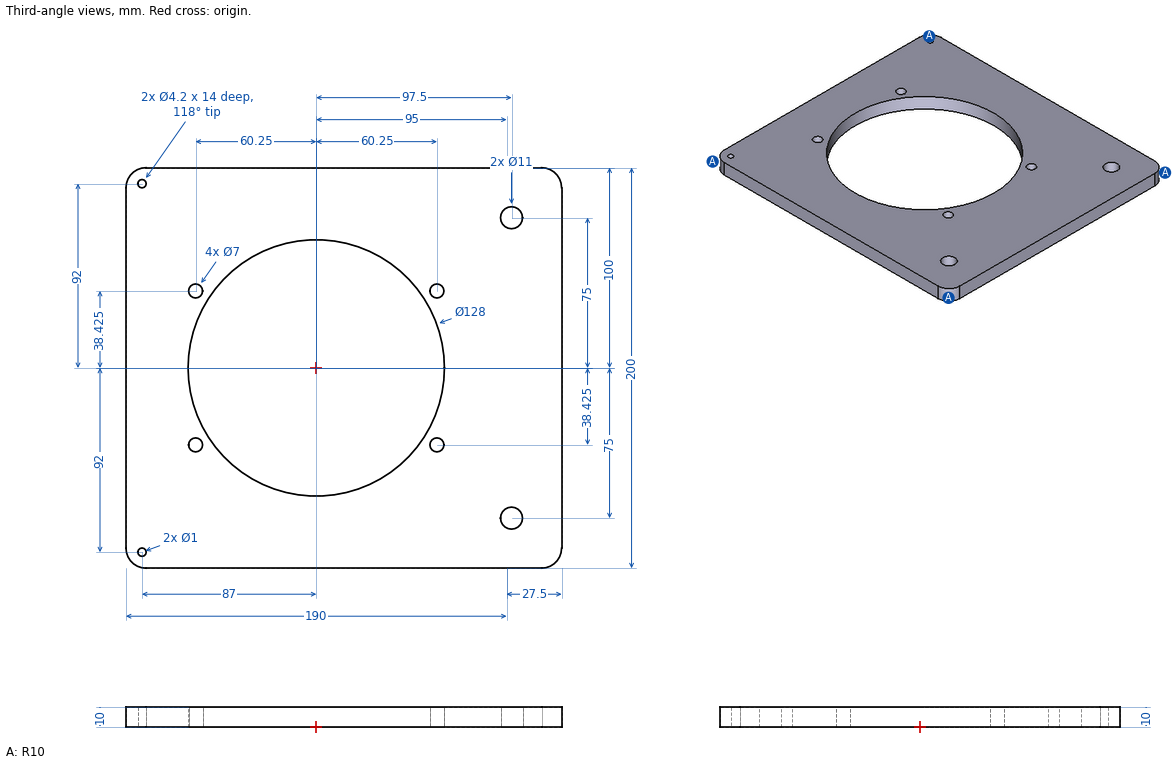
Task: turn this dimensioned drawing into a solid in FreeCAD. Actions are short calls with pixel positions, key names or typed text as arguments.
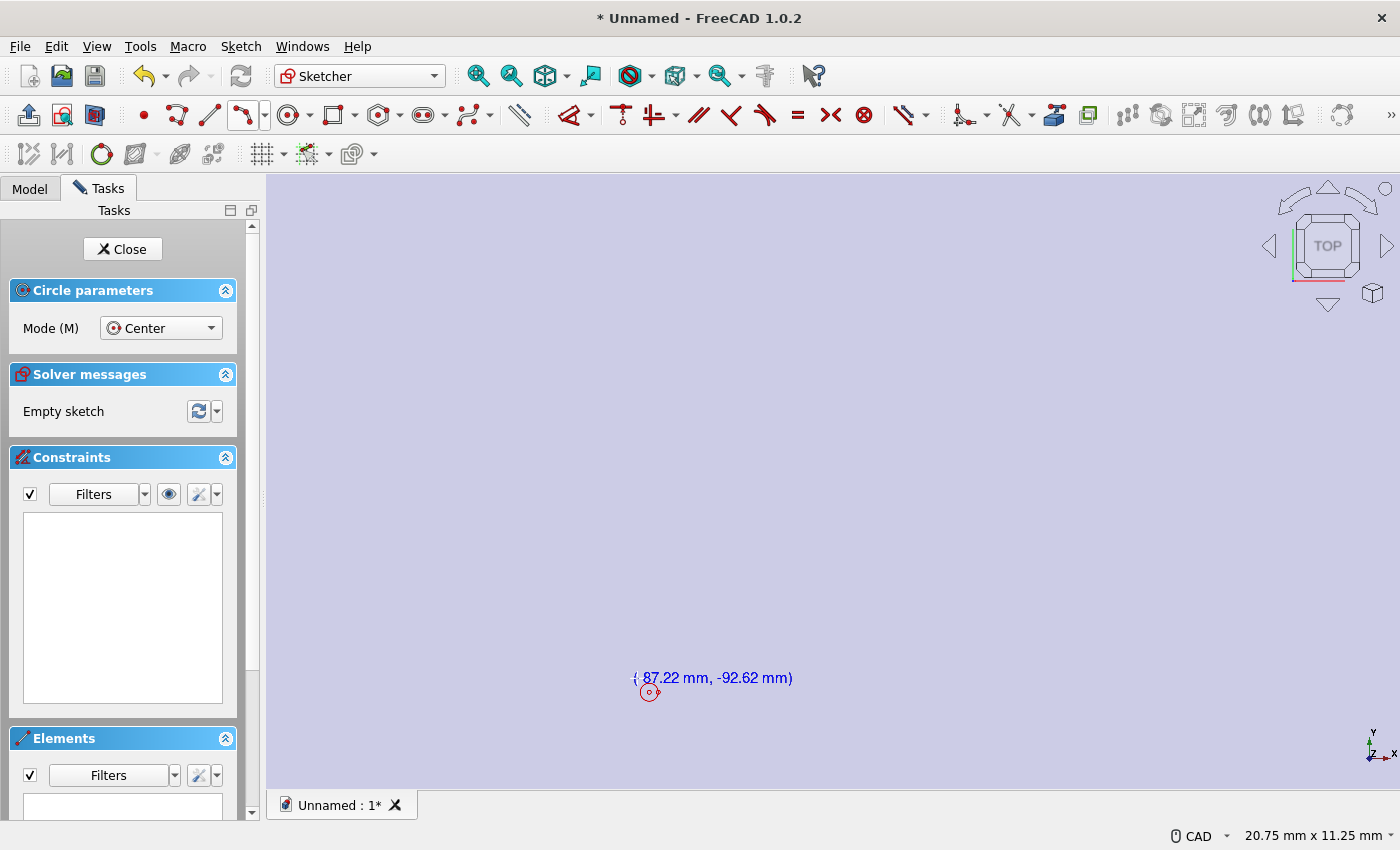
scroll(647, 736, down, 15)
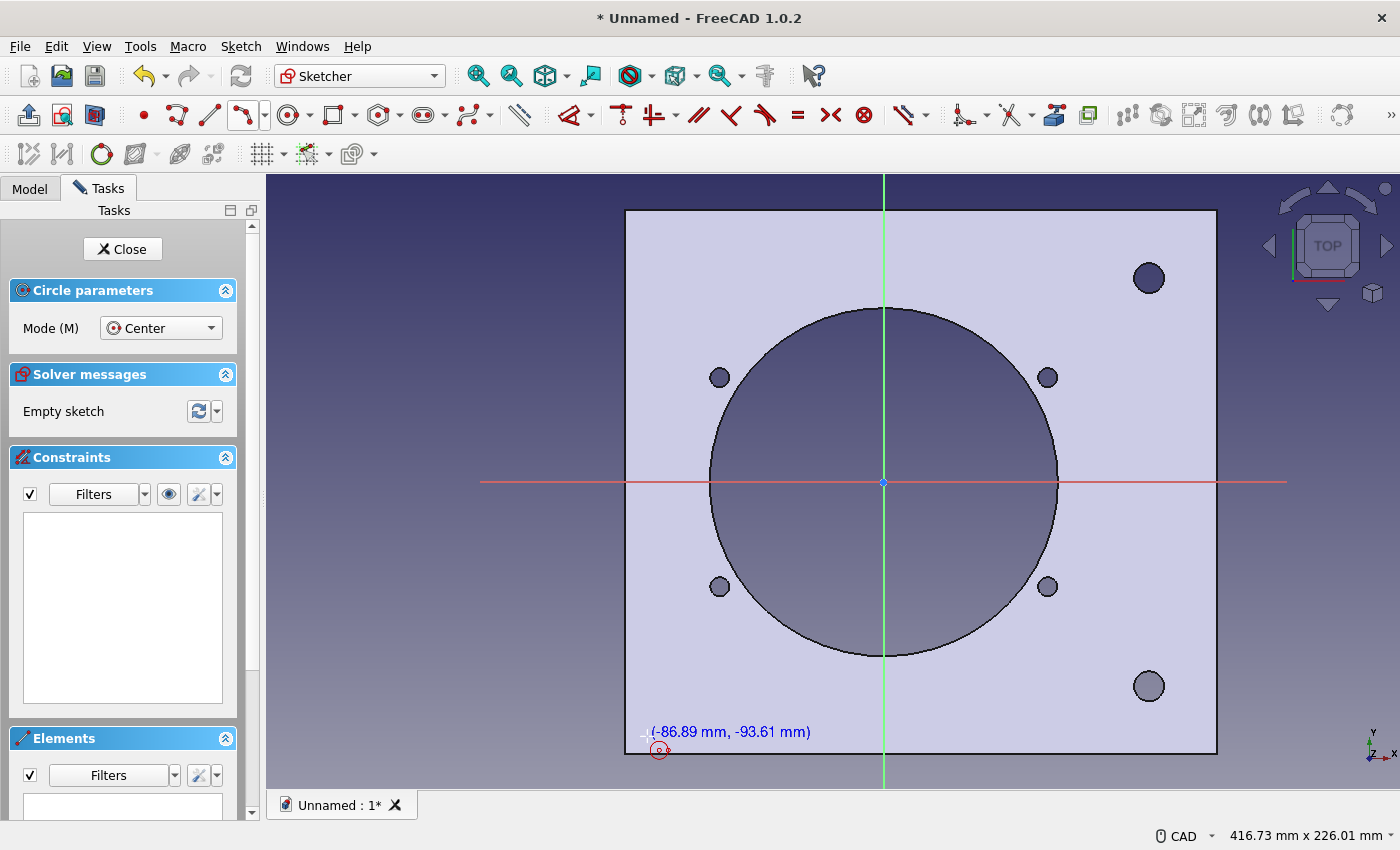
click(647, 733)
move(648, 732)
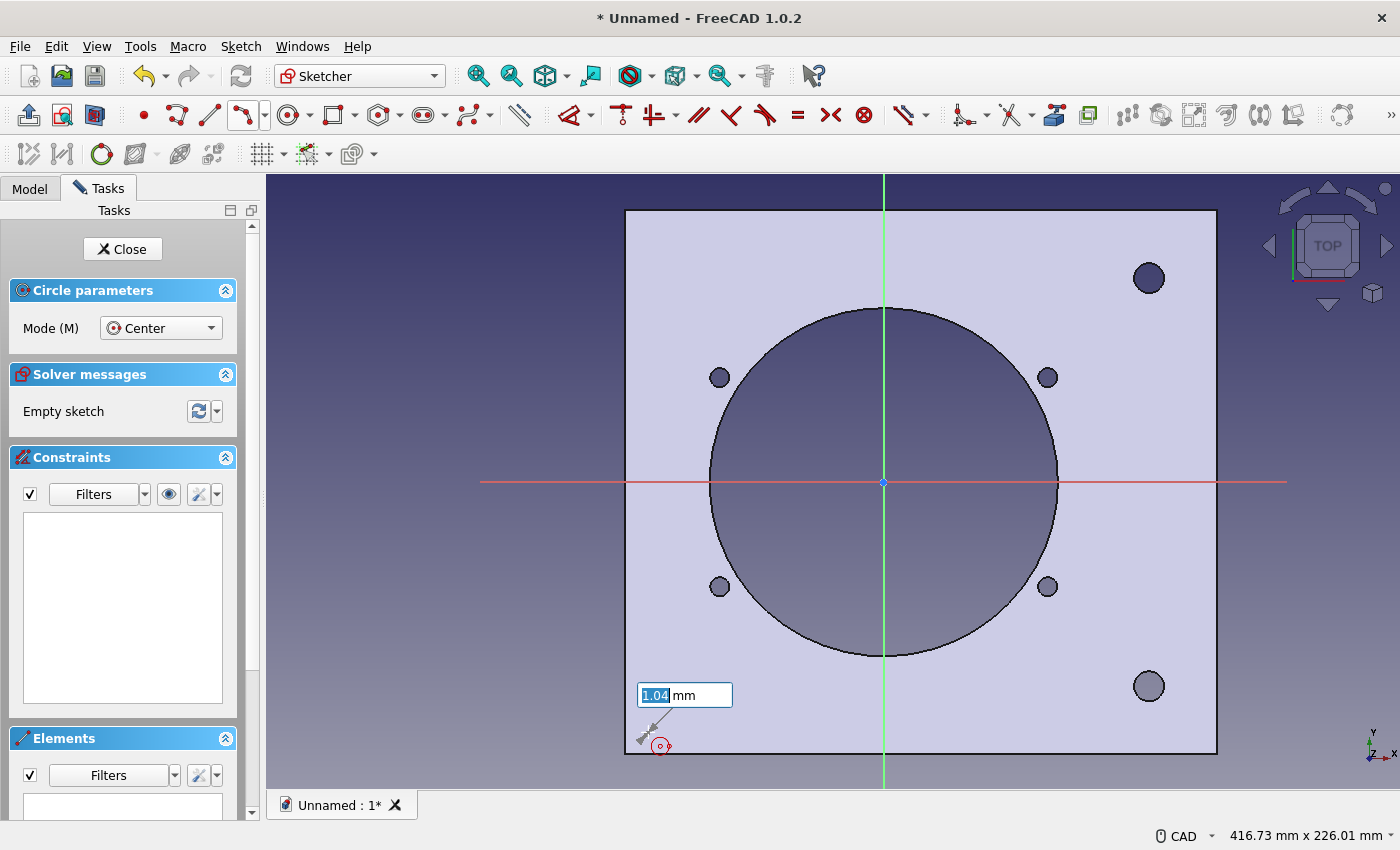
text(1)
key(Return)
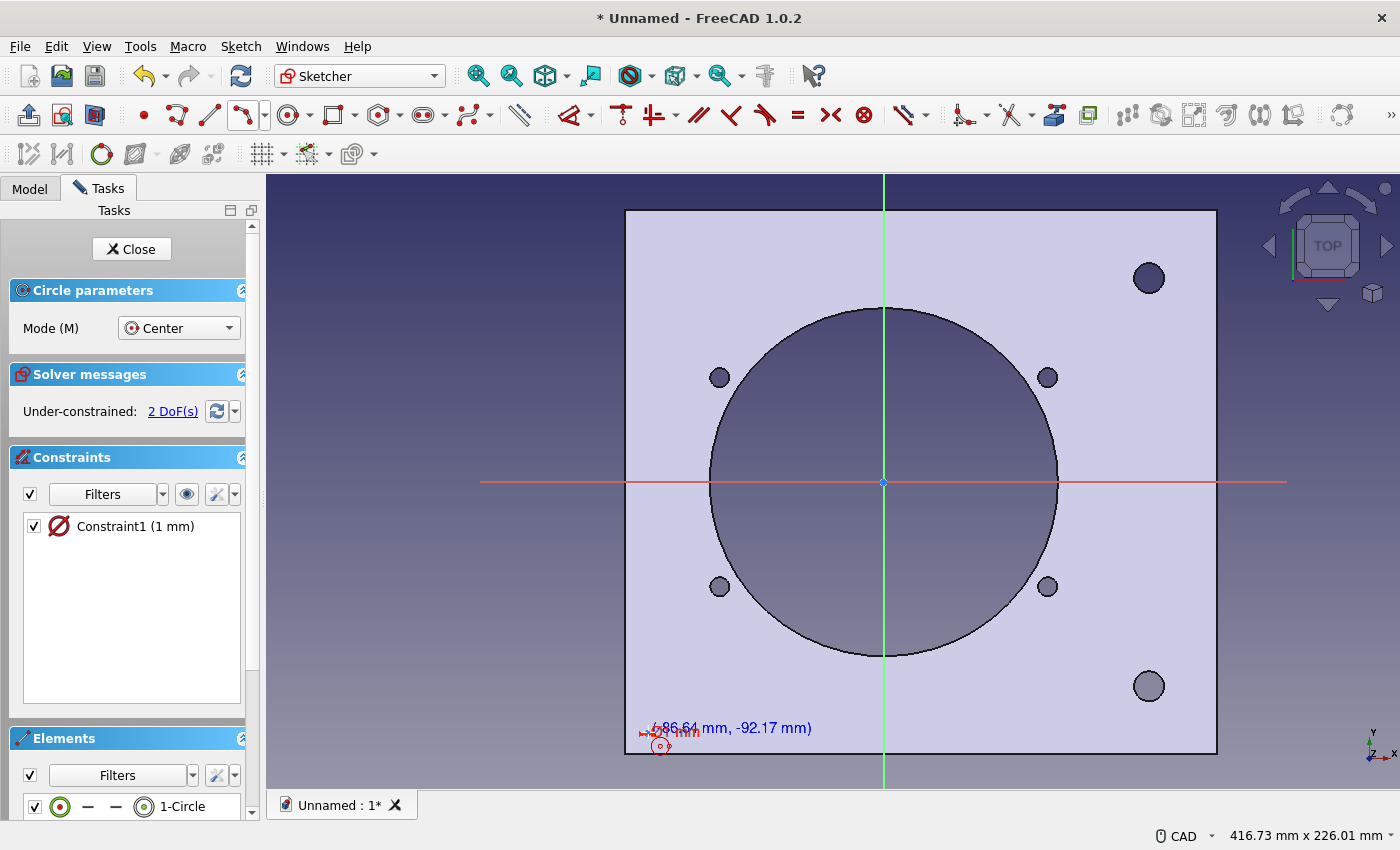
scroll(647, 232, up, 15)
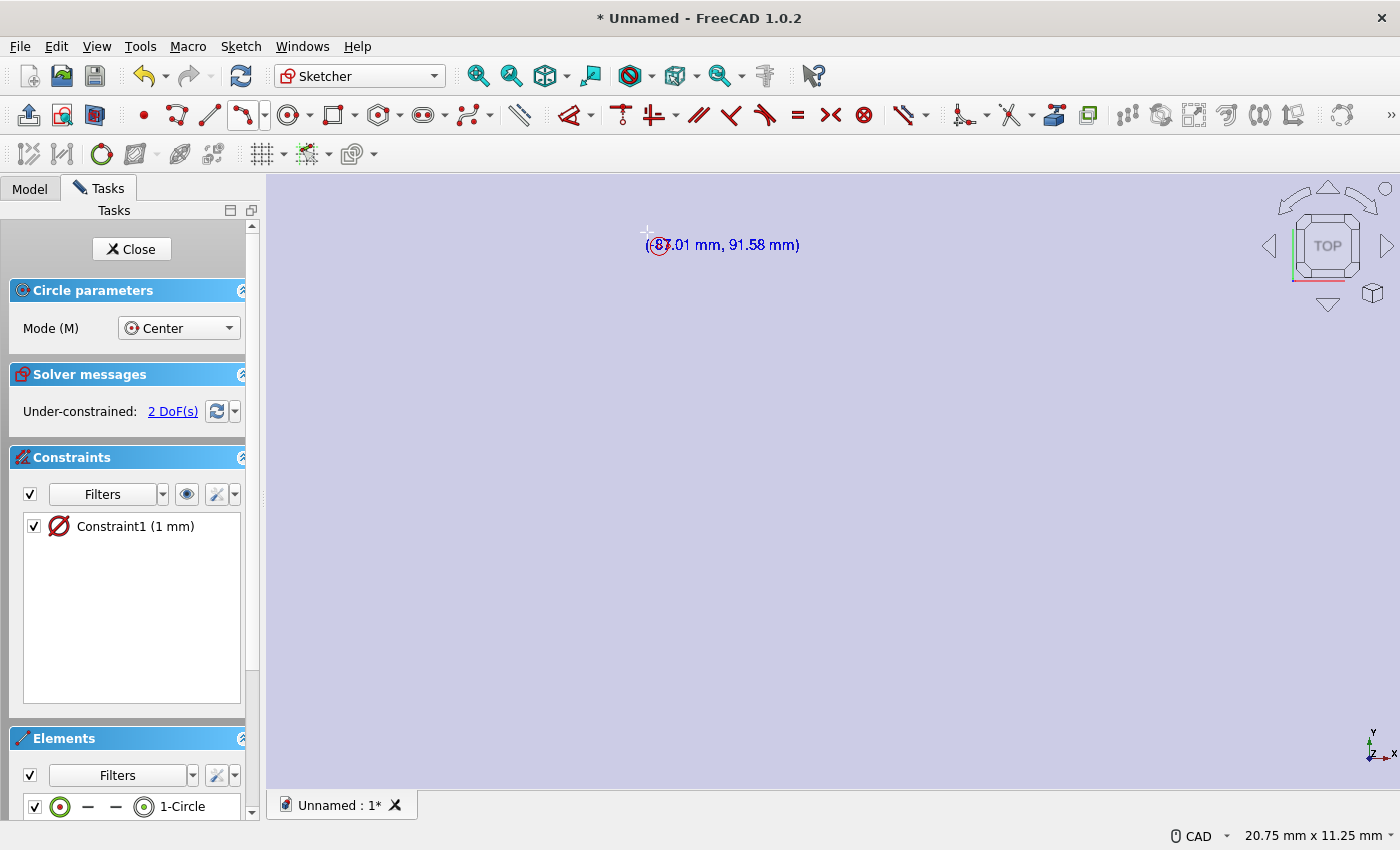
scroll(647, 231, down, 15)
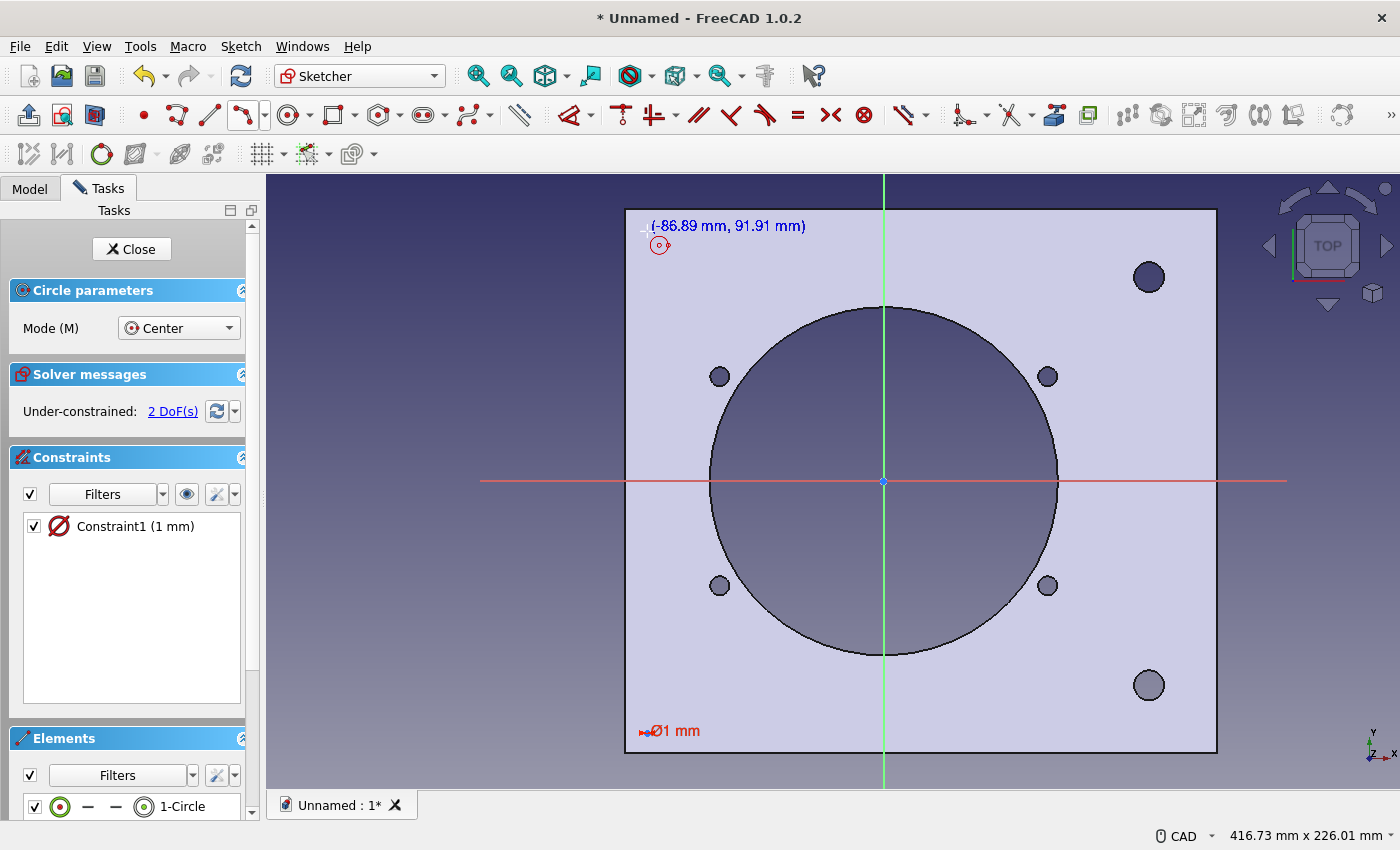
click(647, 231)
move(648, 230)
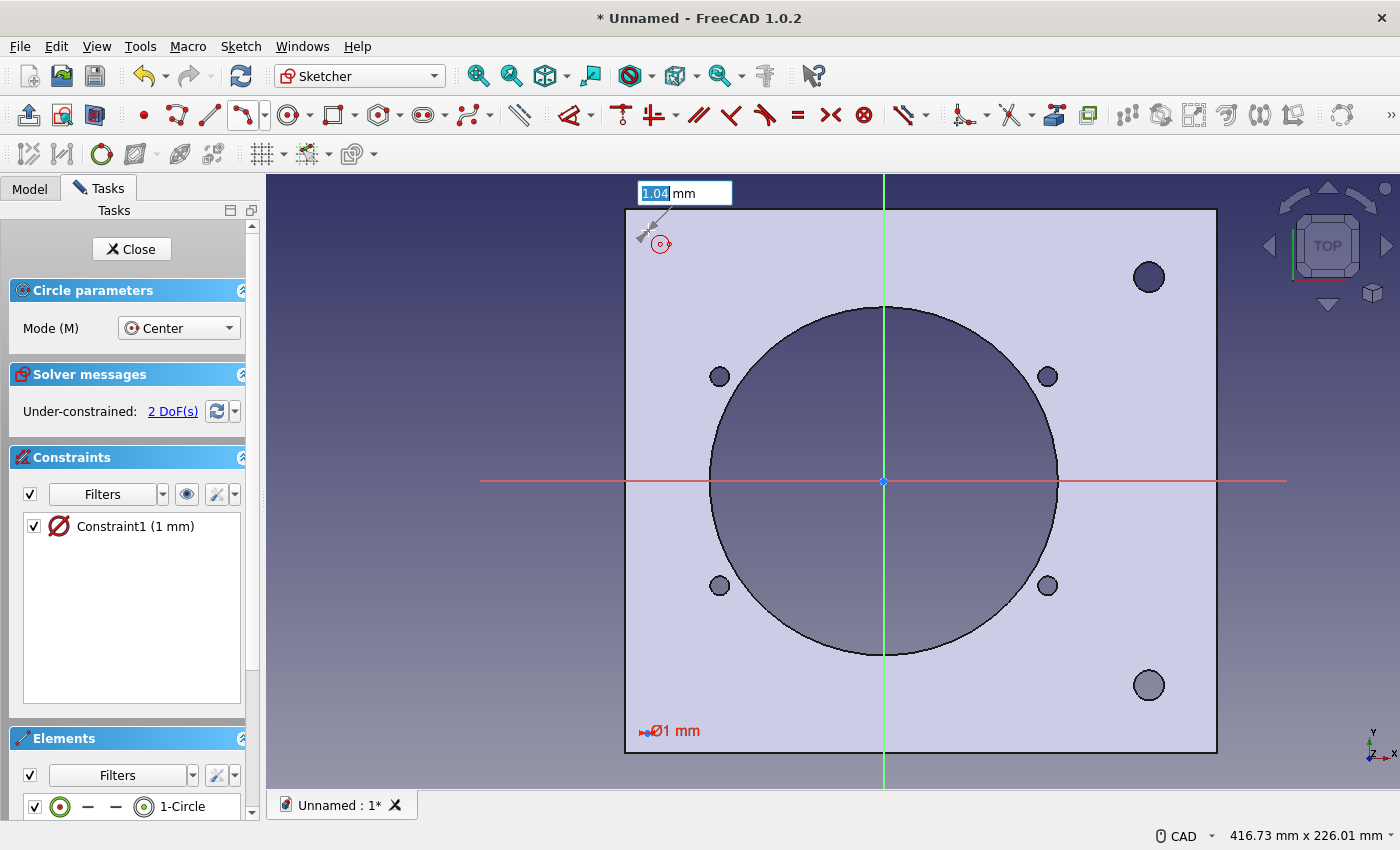
text(1)
key(Return)
key(Escape)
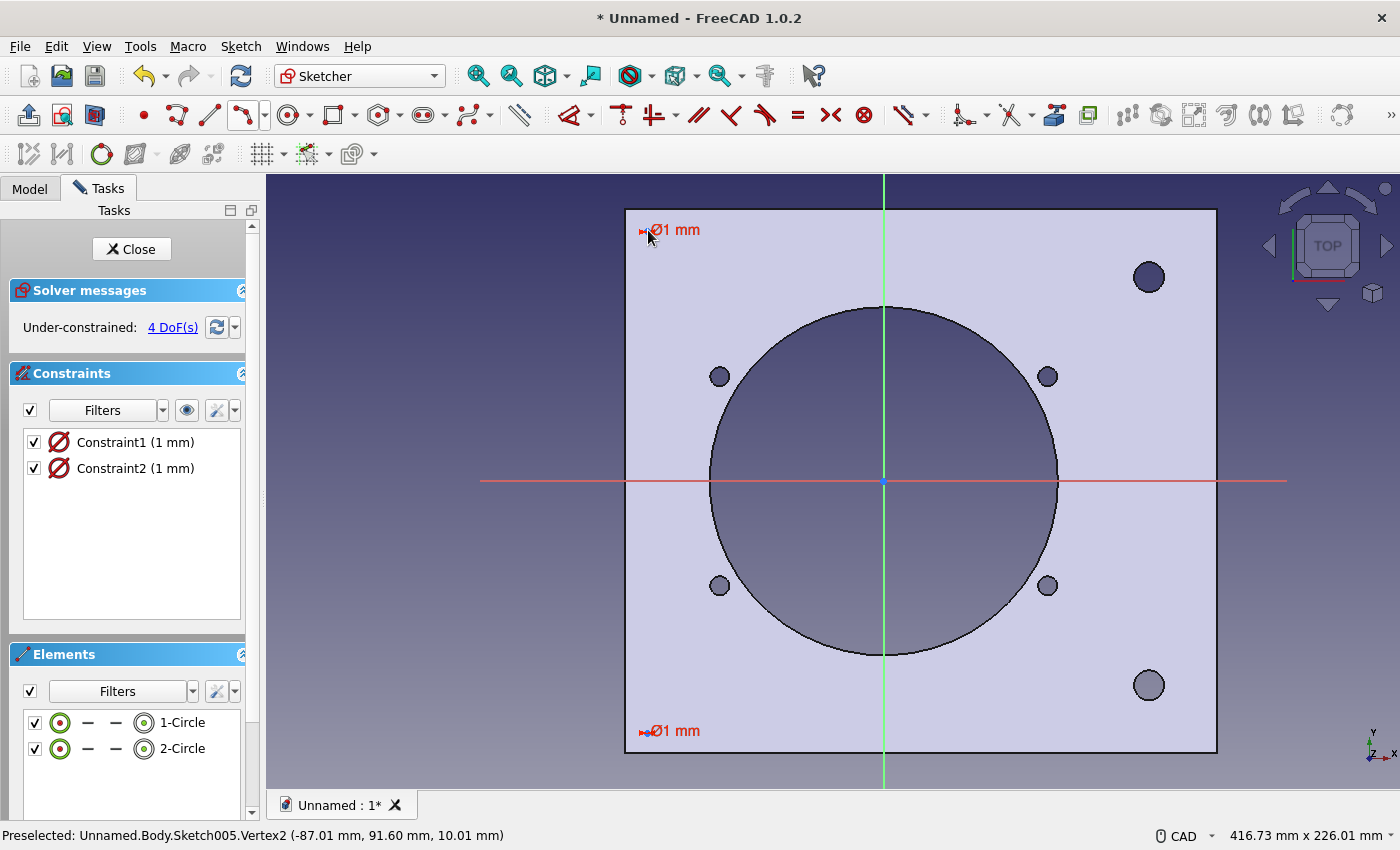
click(647, 733)